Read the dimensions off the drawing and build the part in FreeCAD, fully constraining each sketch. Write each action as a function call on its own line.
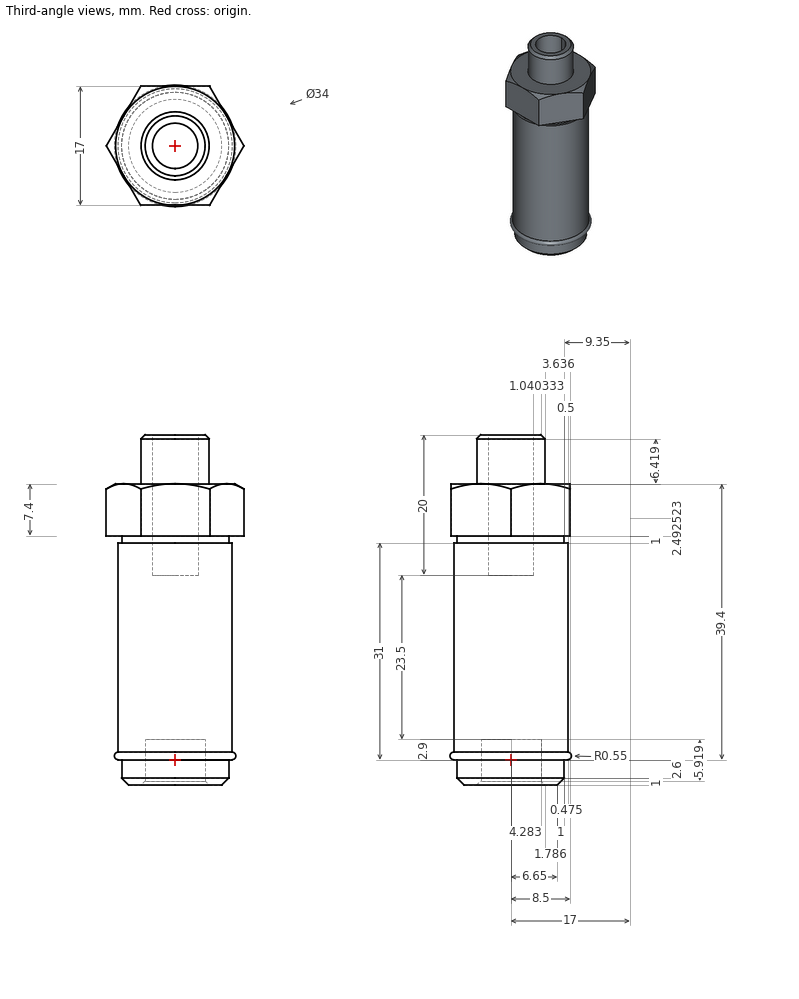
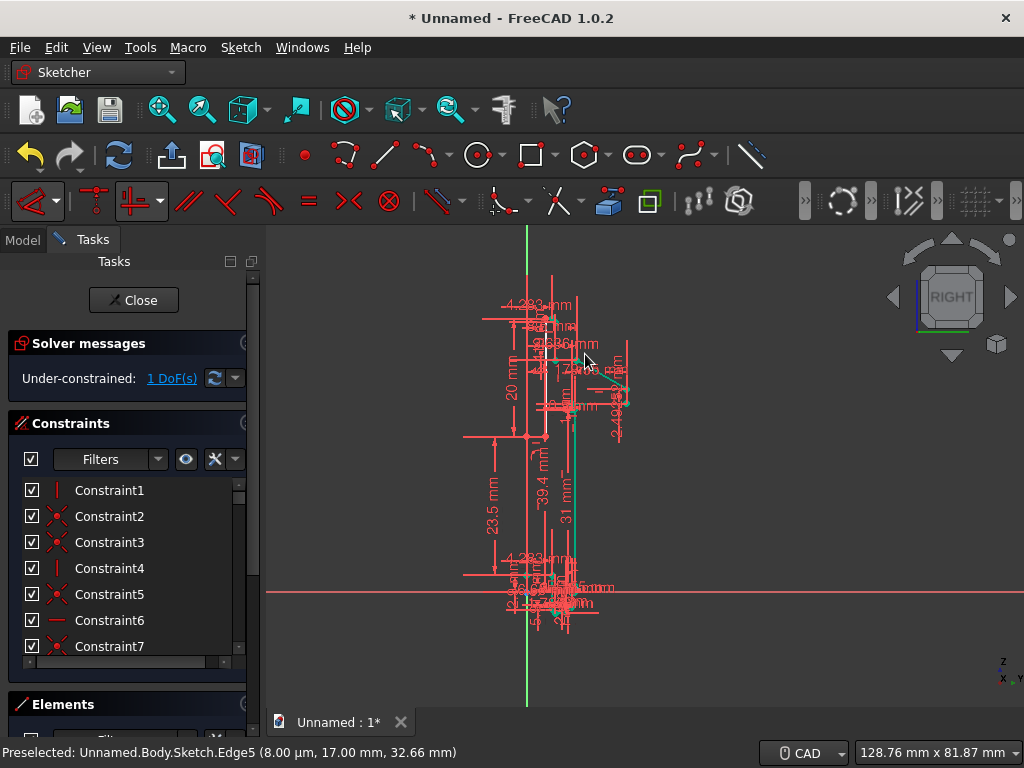
scroll(550, 319, up, 10)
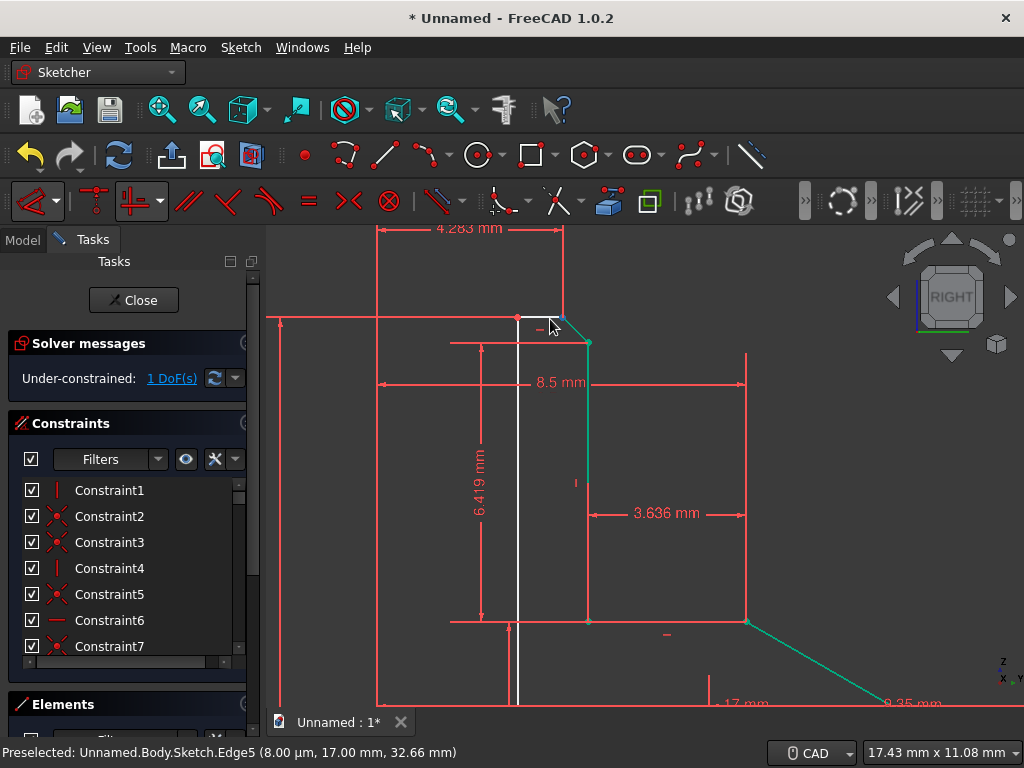
click(545, 317)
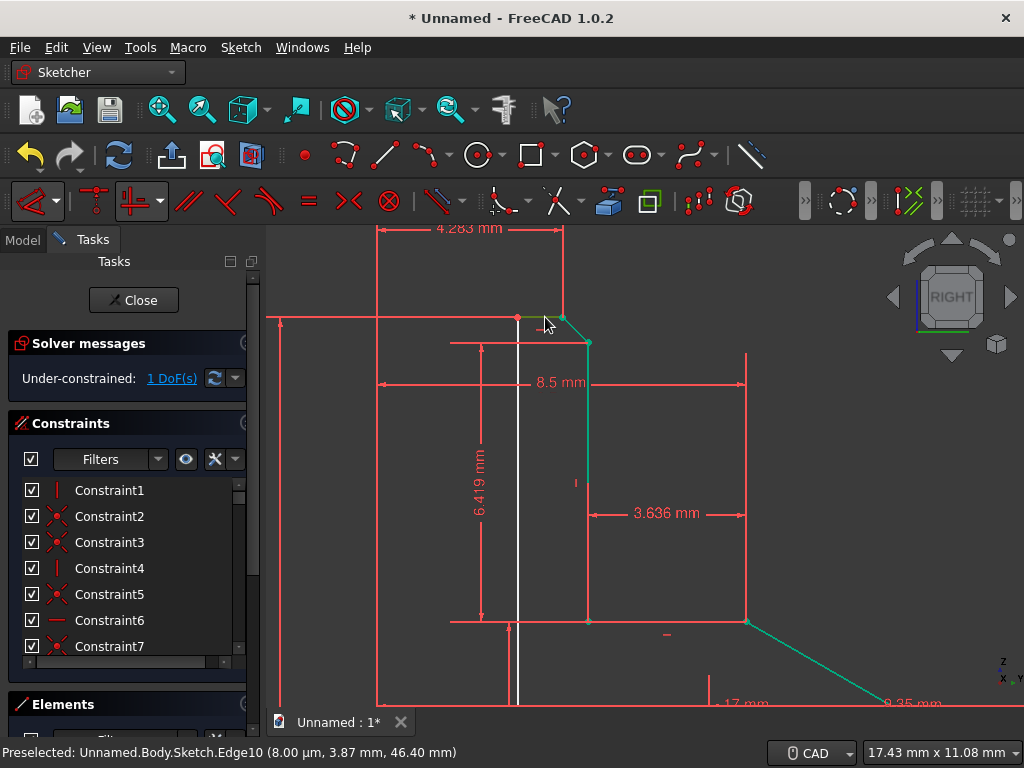
click(58, 202)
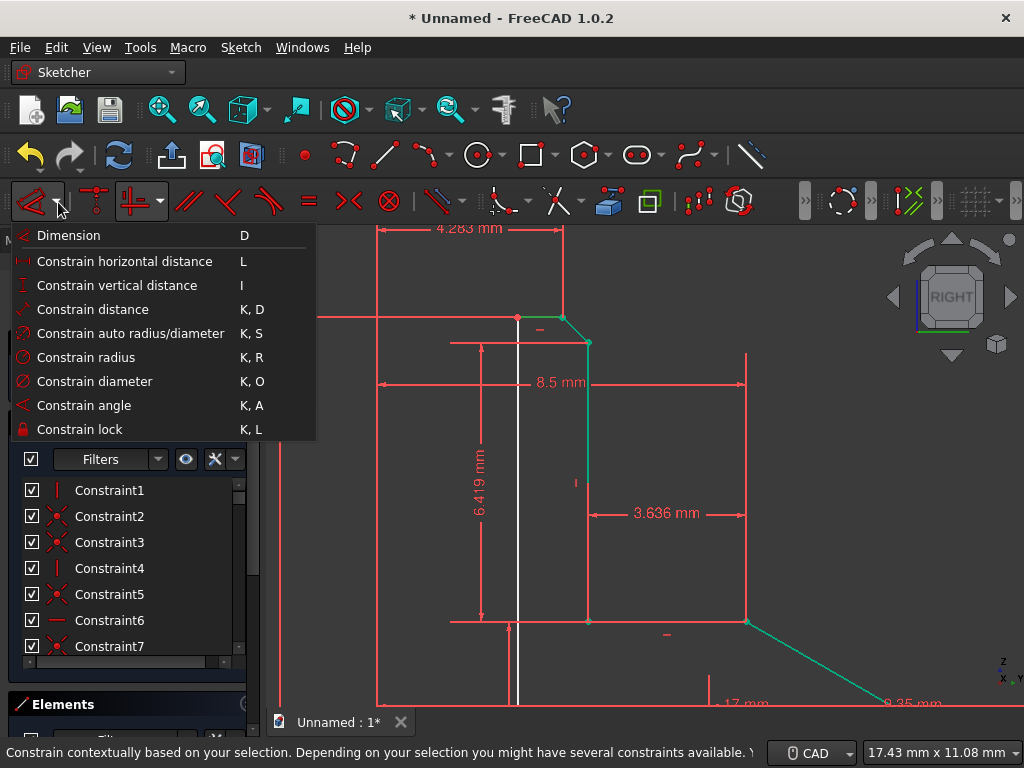
click(164, 261)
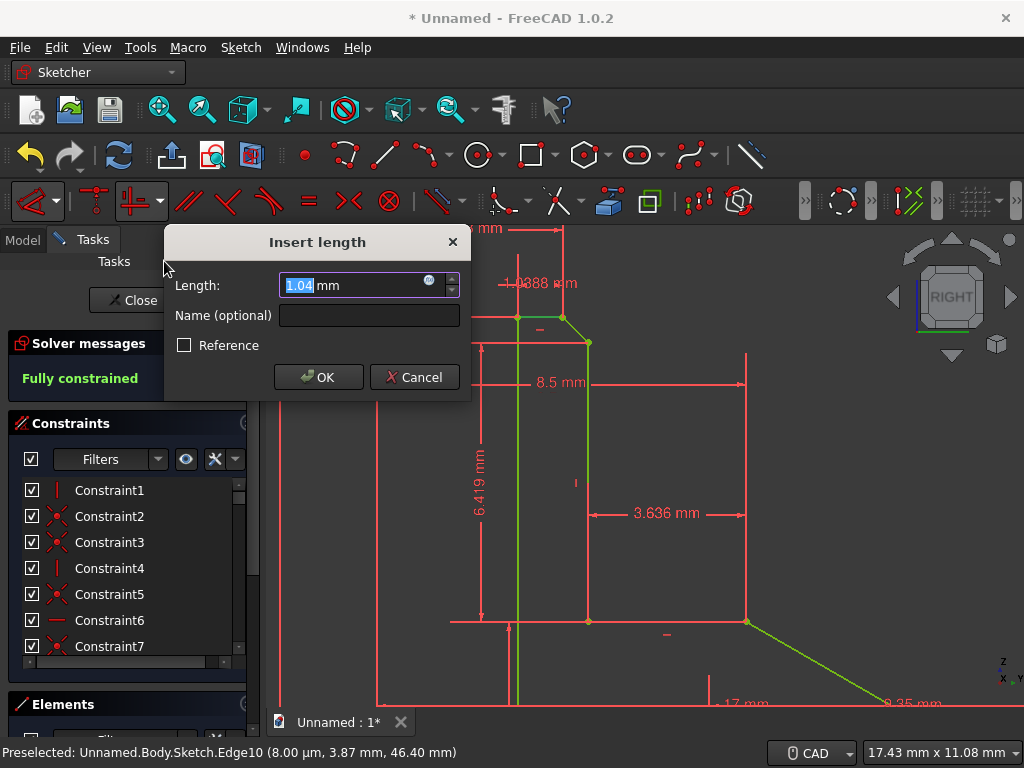
text(1.040333)
key(Return)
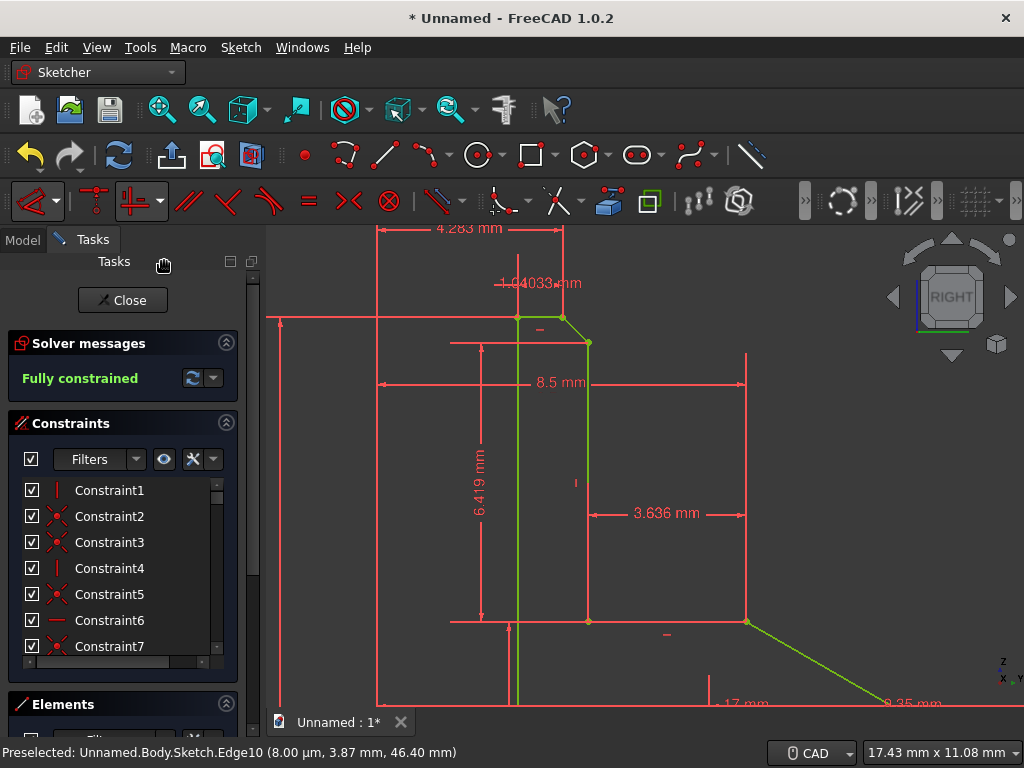
click(123, 300)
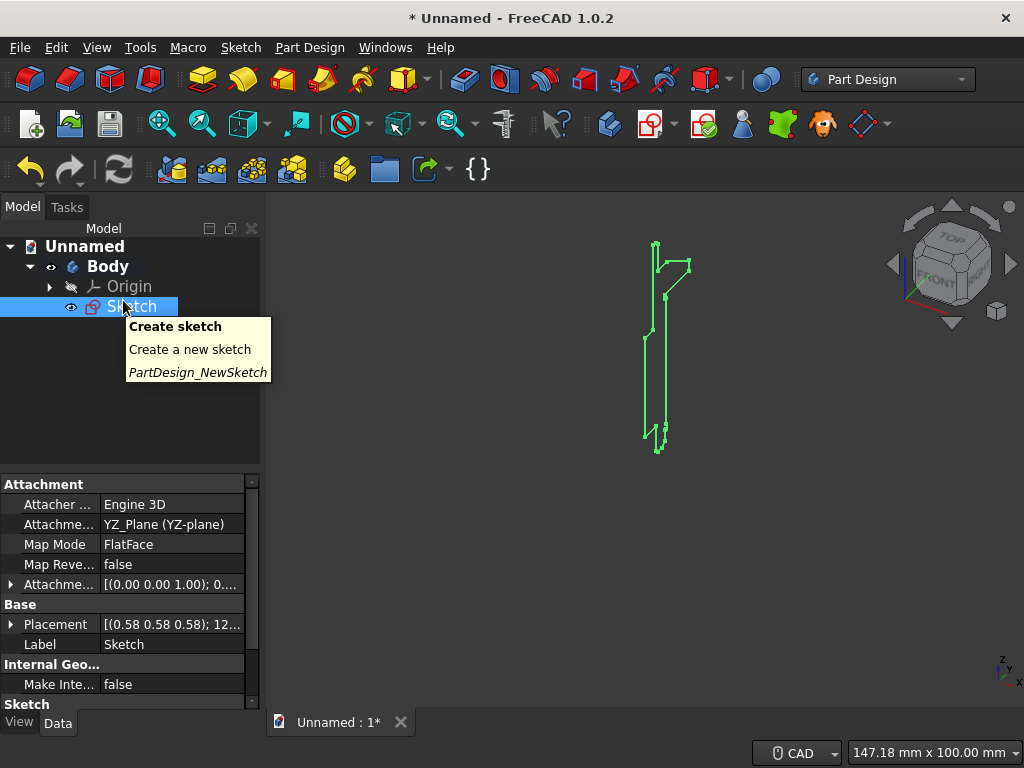
click(244, 80)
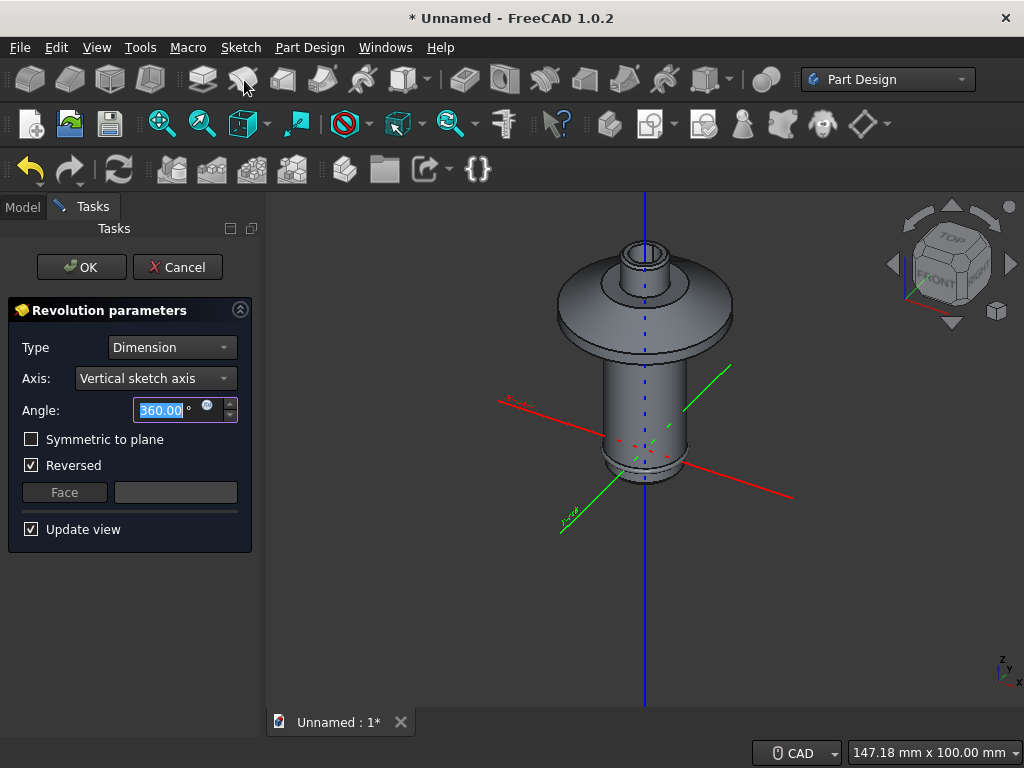
click(82, 267)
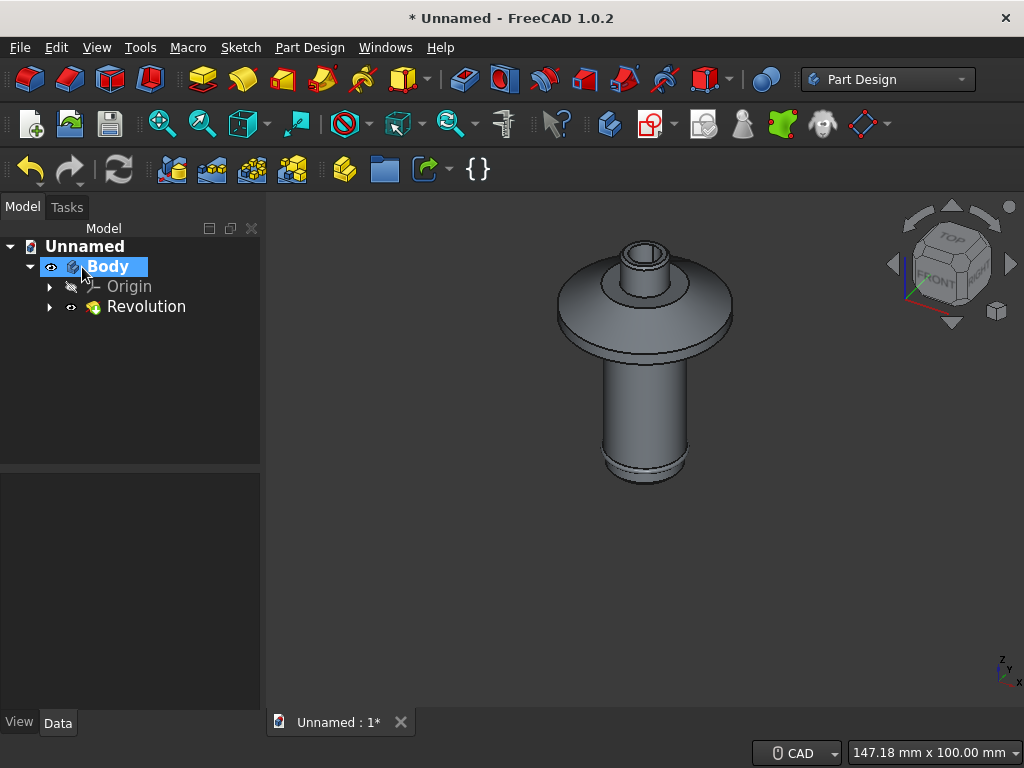
key(v)
key(f)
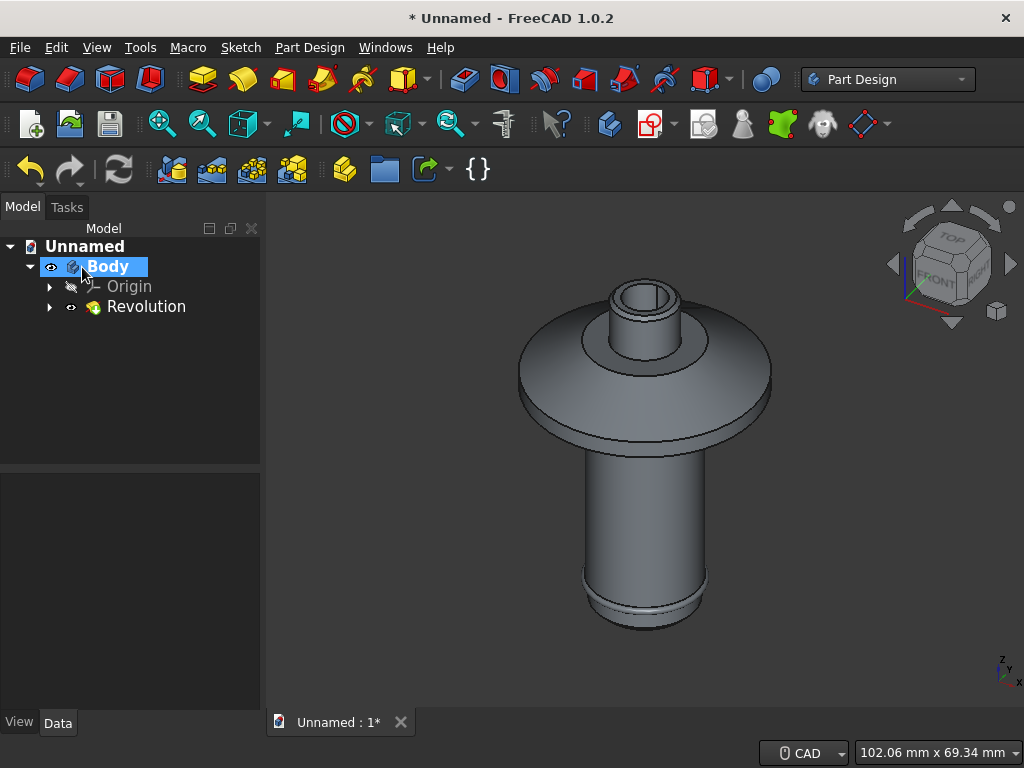
key(5)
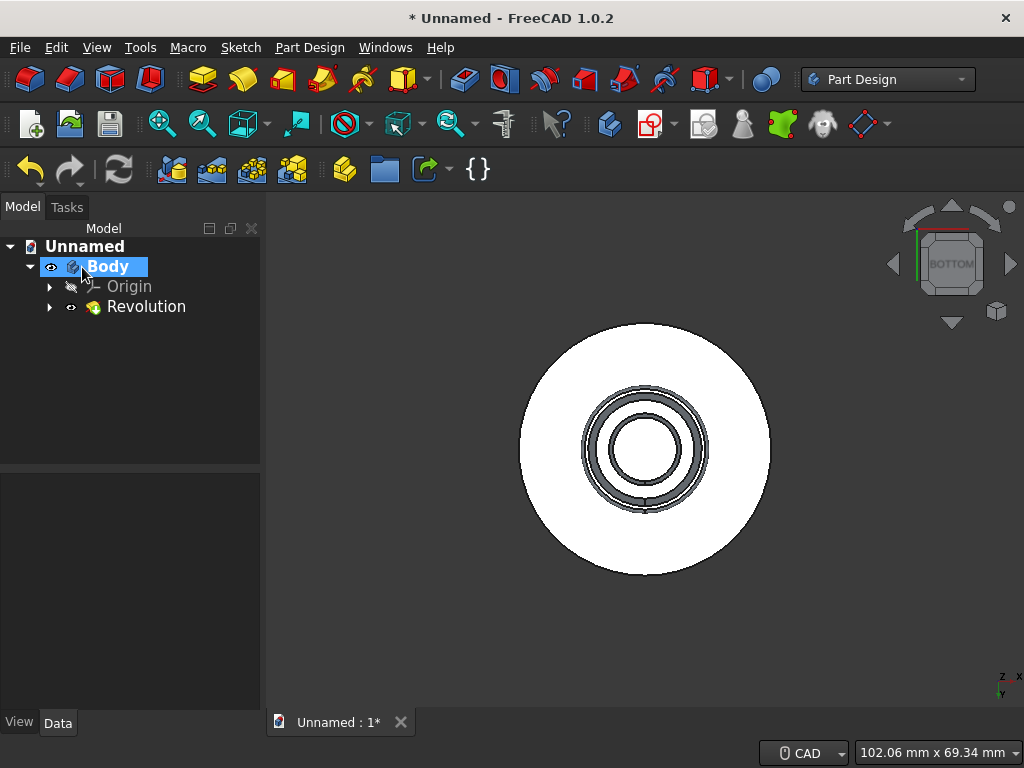
click(573, 376)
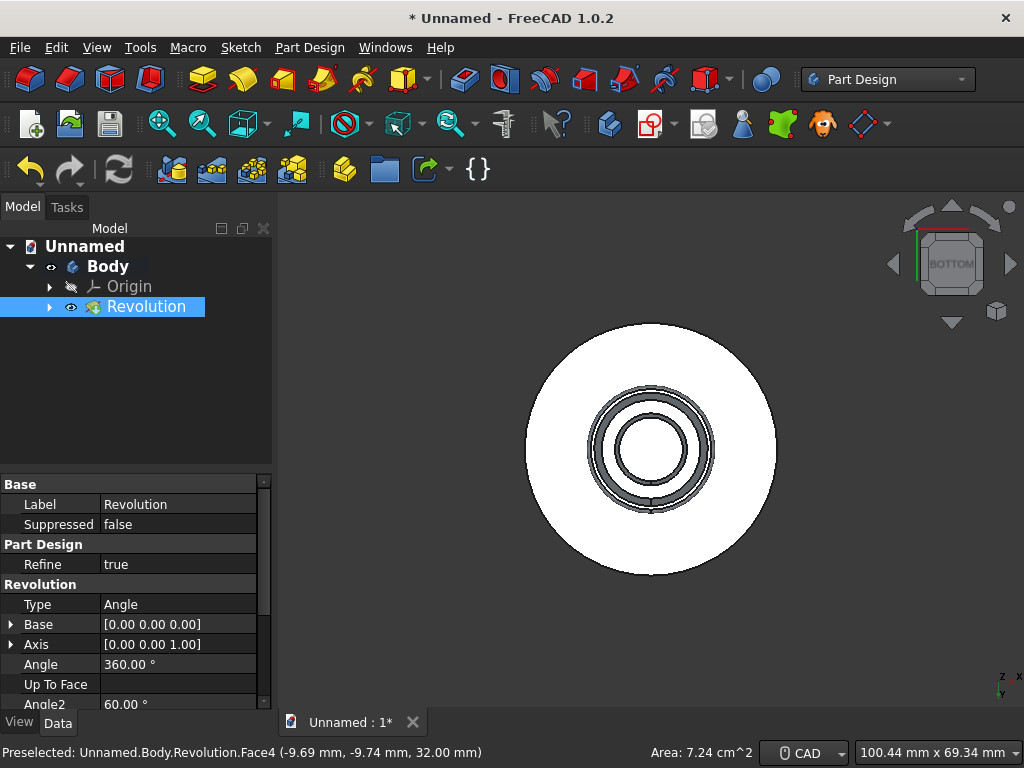
click(650, 124)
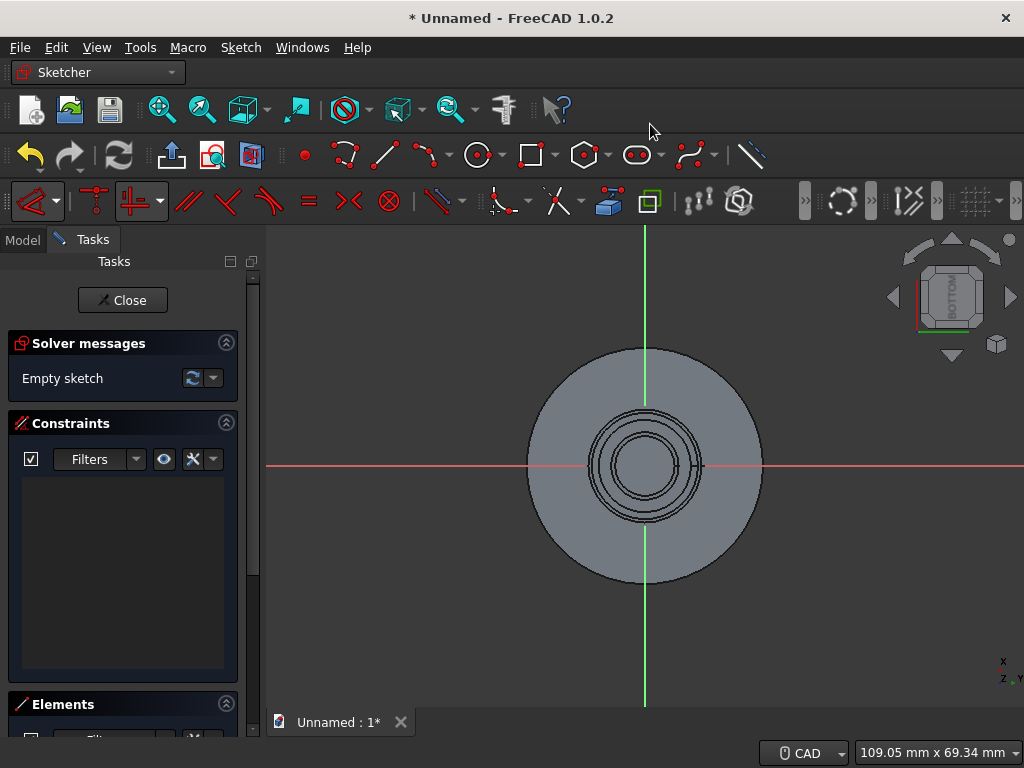
key(g)
key(p)
key(6)